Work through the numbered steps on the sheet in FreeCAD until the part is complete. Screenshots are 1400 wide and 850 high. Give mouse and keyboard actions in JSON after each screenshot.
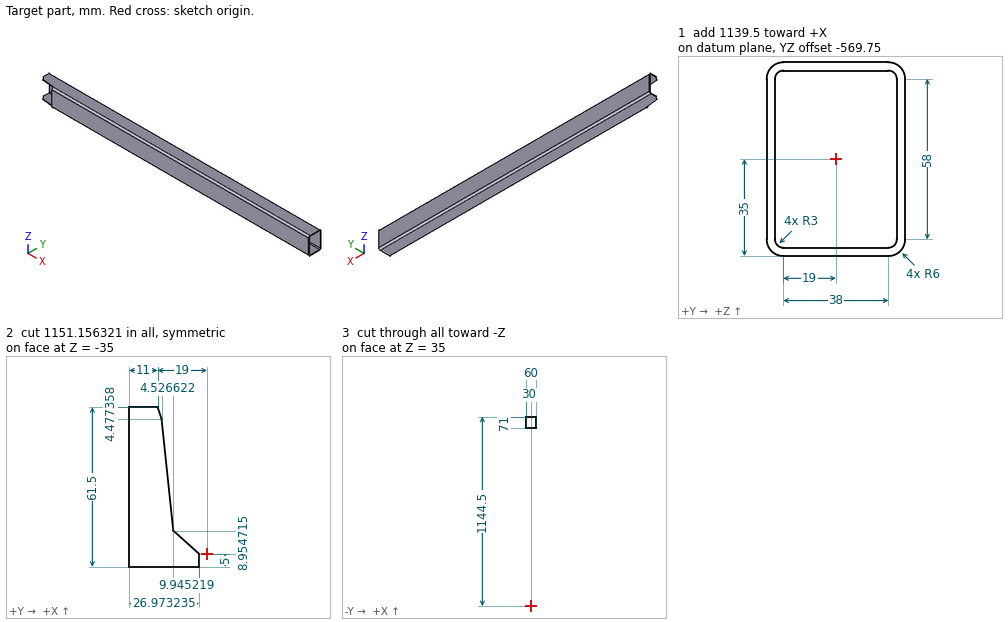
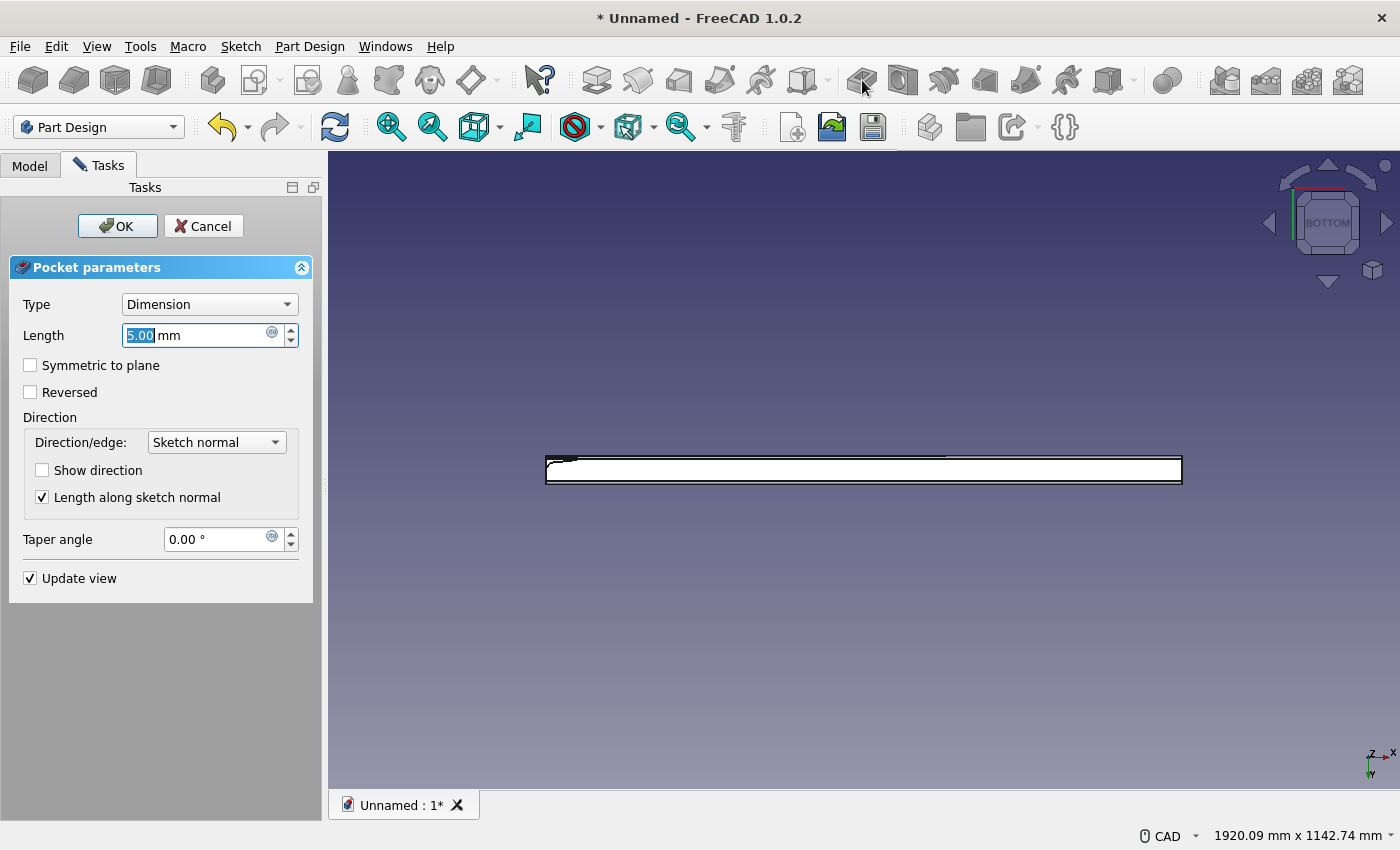
{"action": "type", "text": "1151.156321"}
{"action": "key", "text": "Tab"}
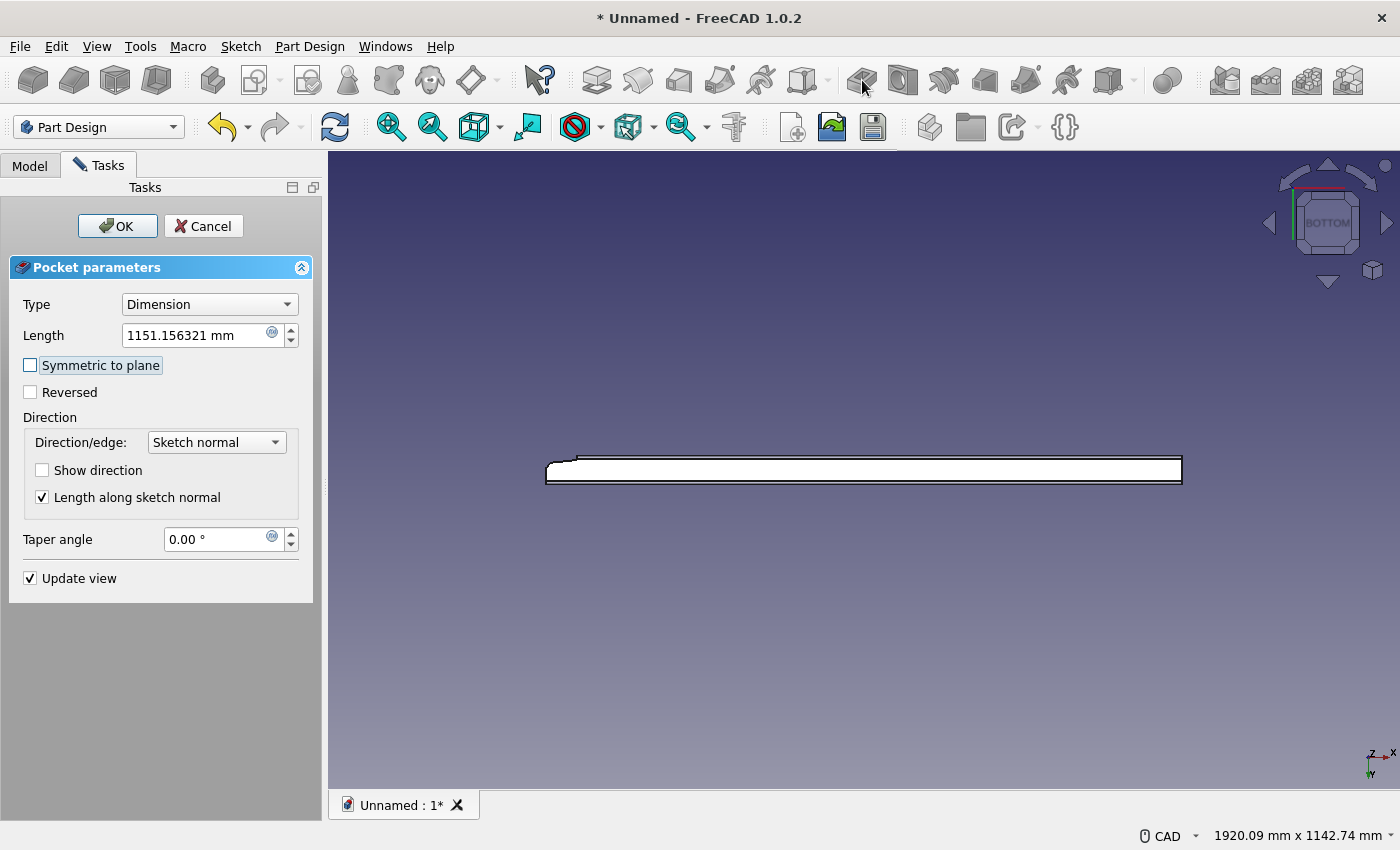
{"action": "left_click", "coordinate": [31, 365]}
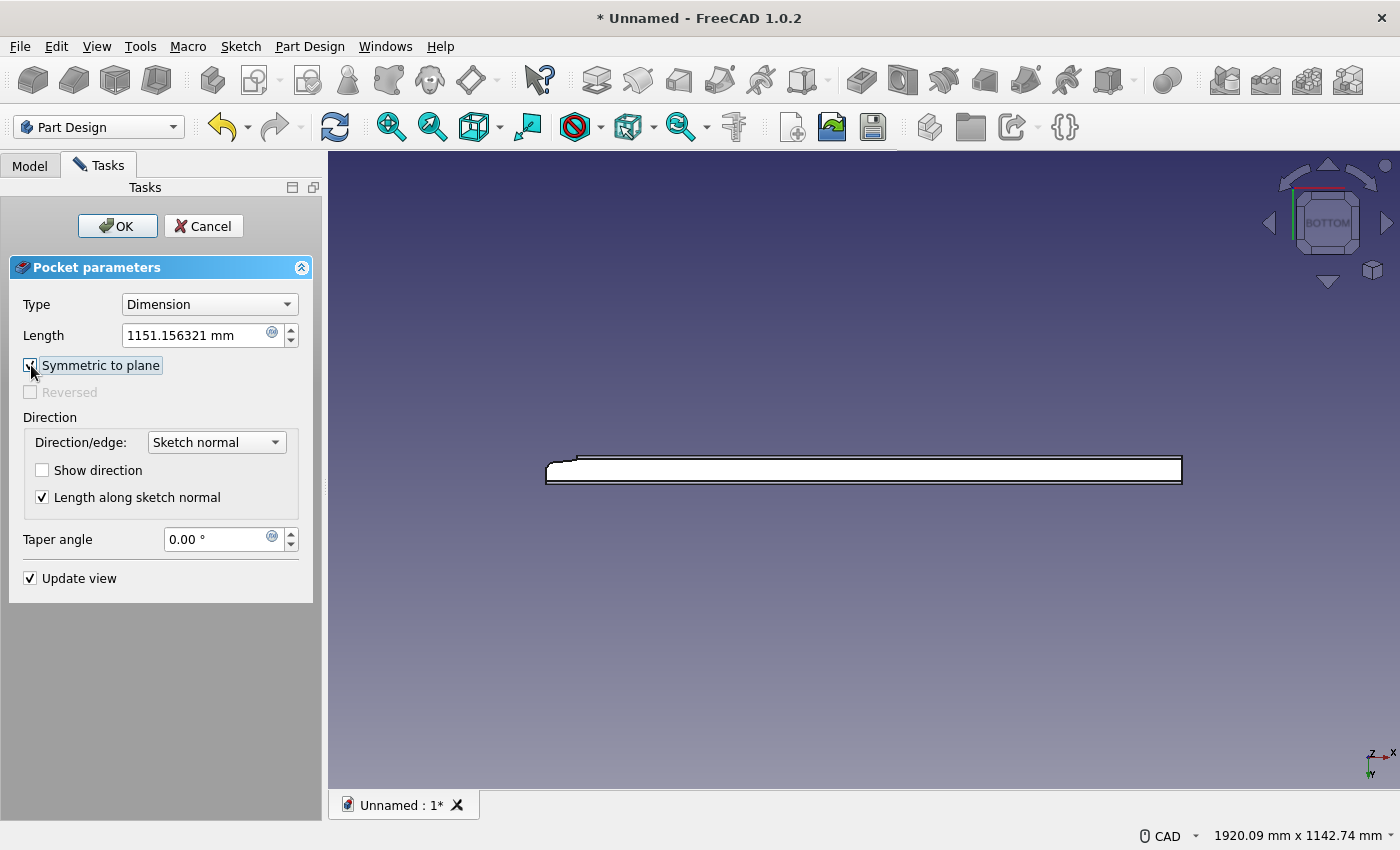
{"action": "left_click", "coordinate": [118, 226]}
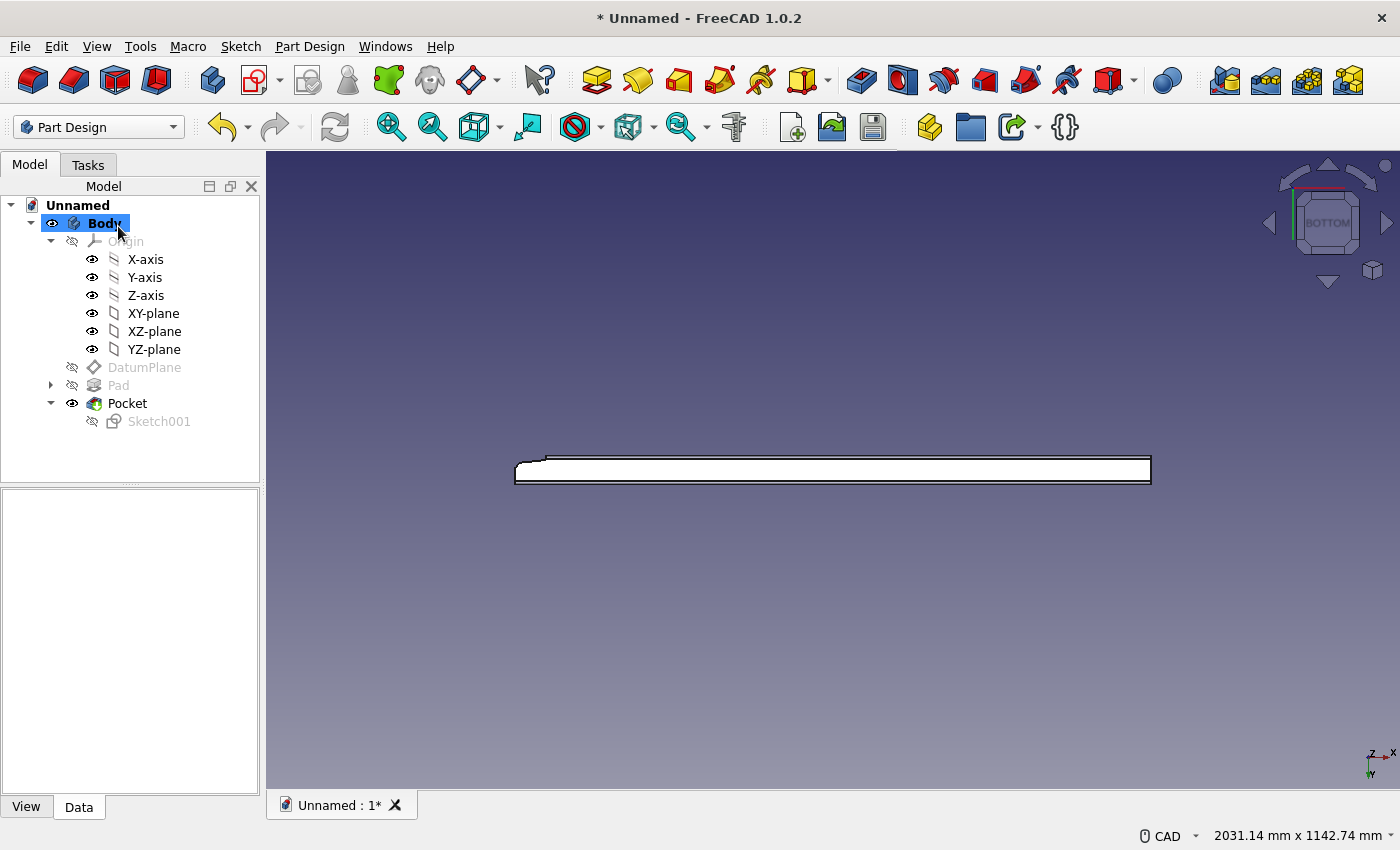
{"action": "key", "text": "0"}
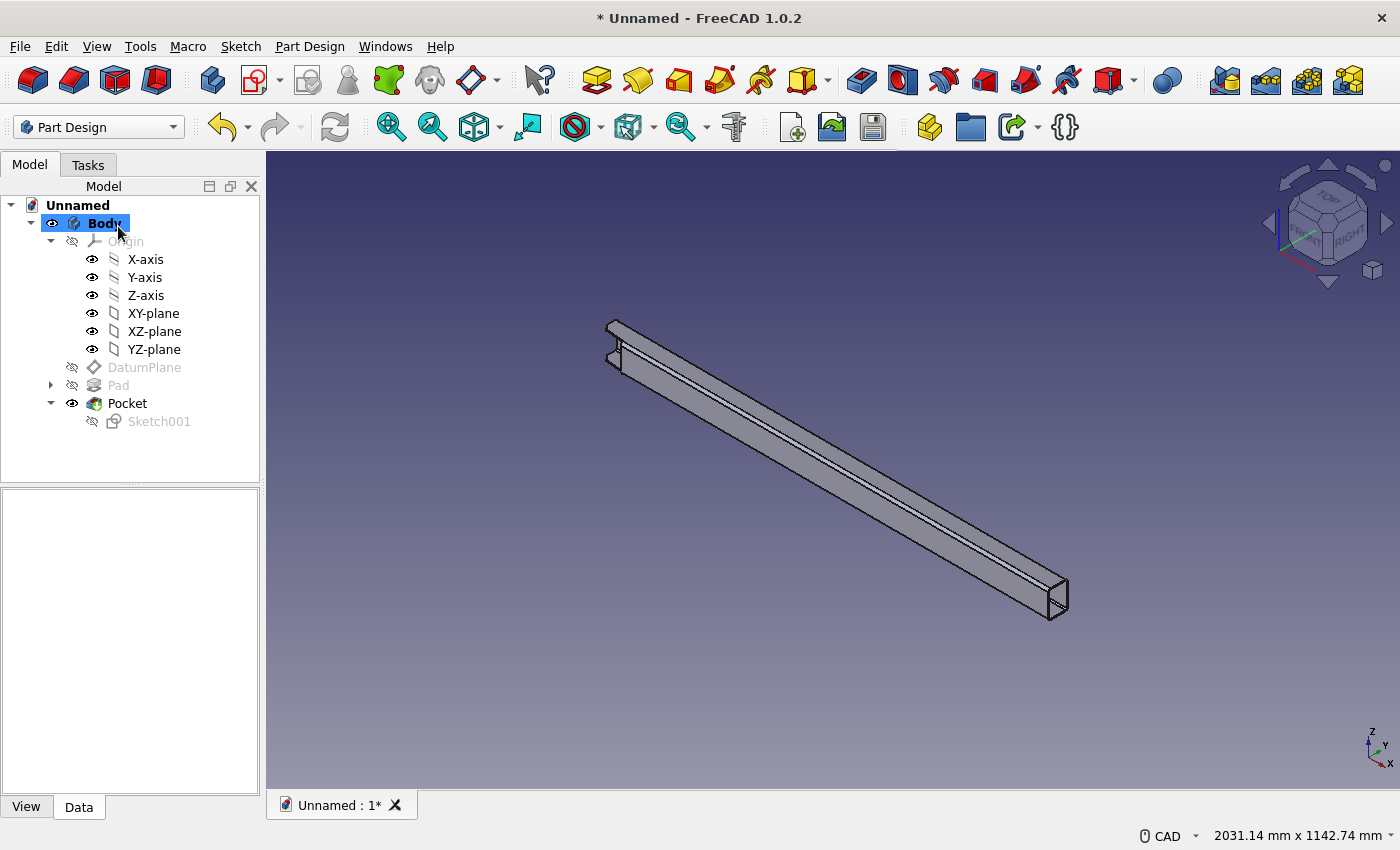
{"action": "left_click", "coordinate": [1028, 563]}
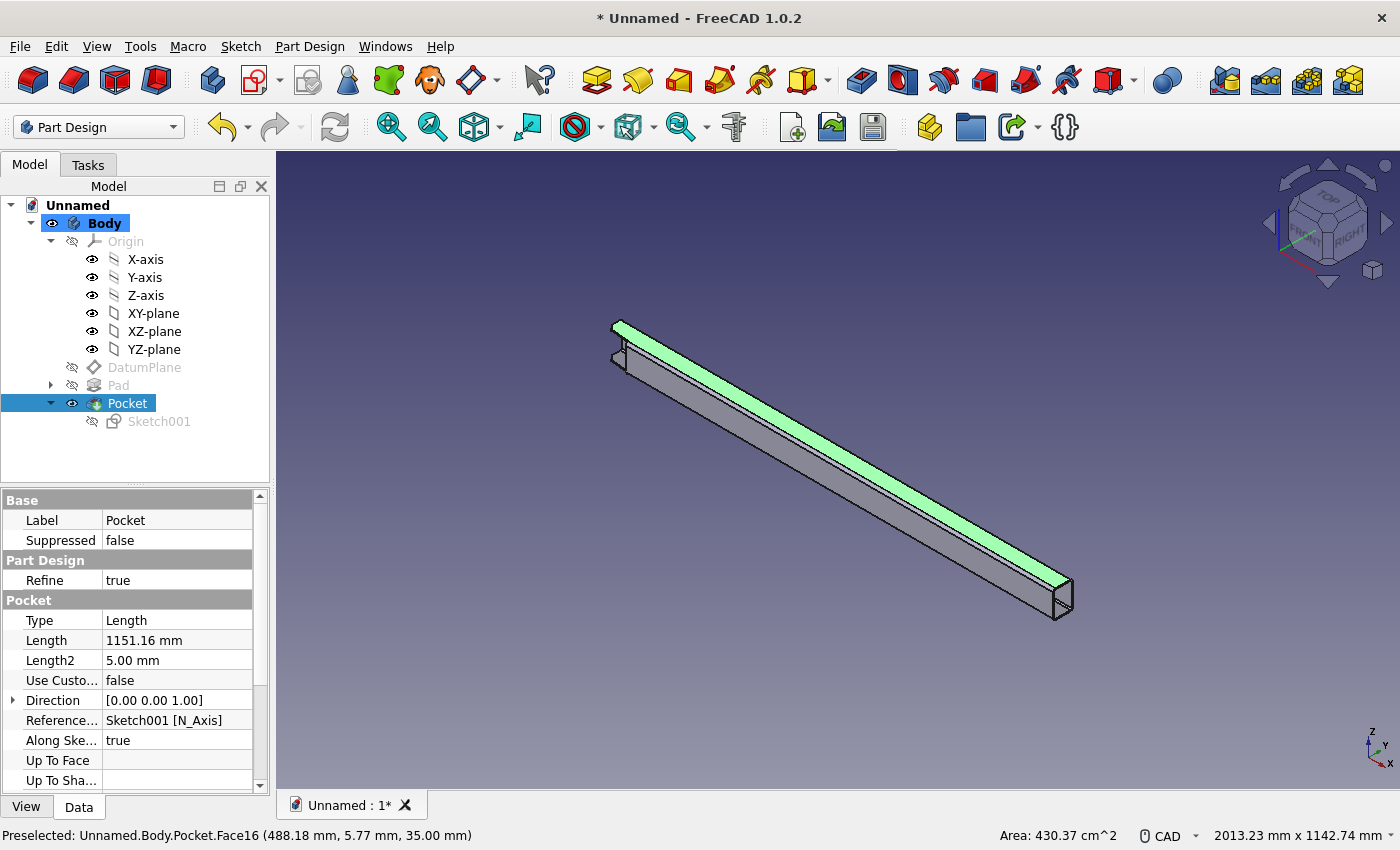
{"action": "left_click", "coordinate": [254, 80]}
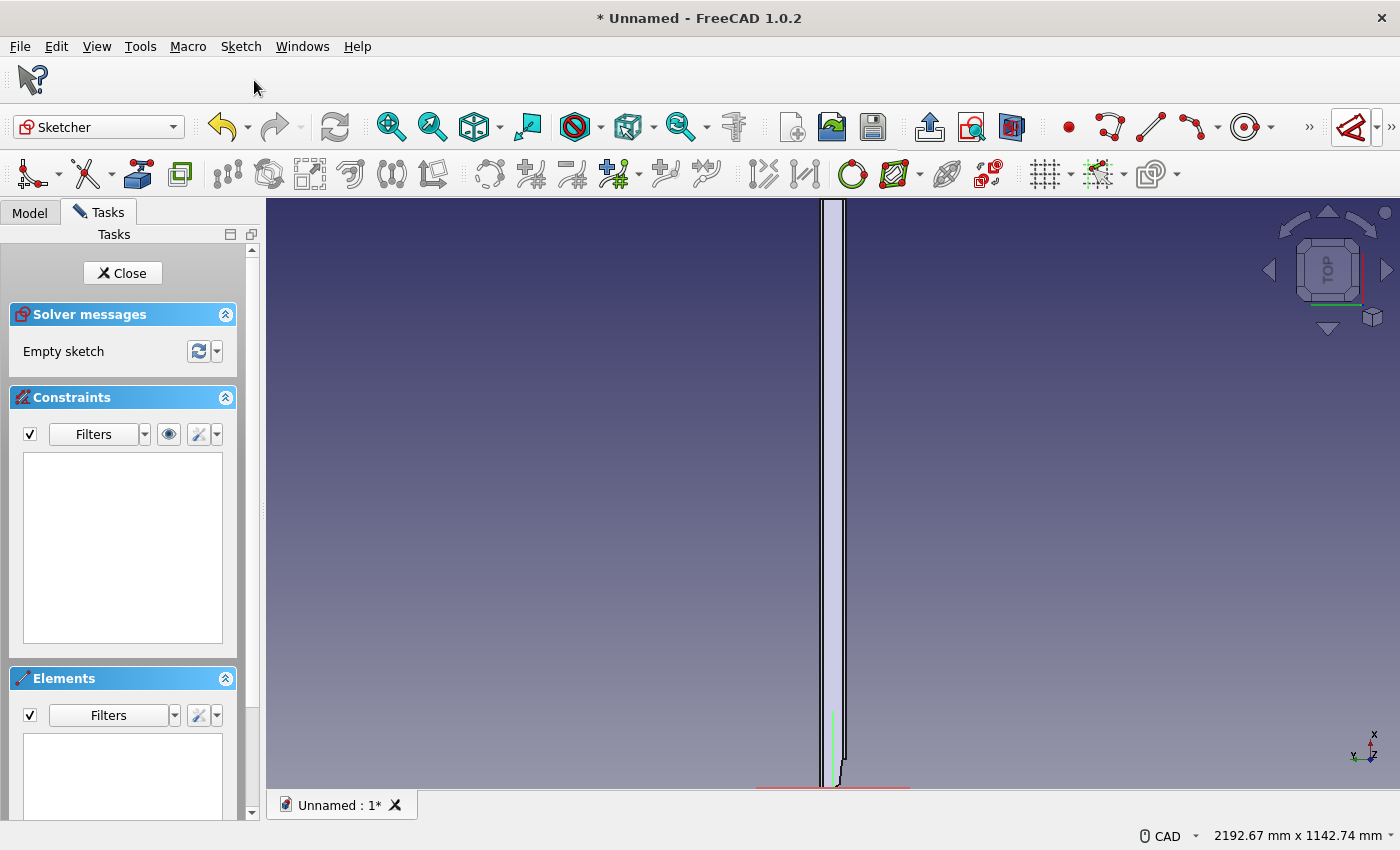
{"action": "scroll", "coordinate": [764, 494], "scroll_direction": "down", "scroll_amount": 5}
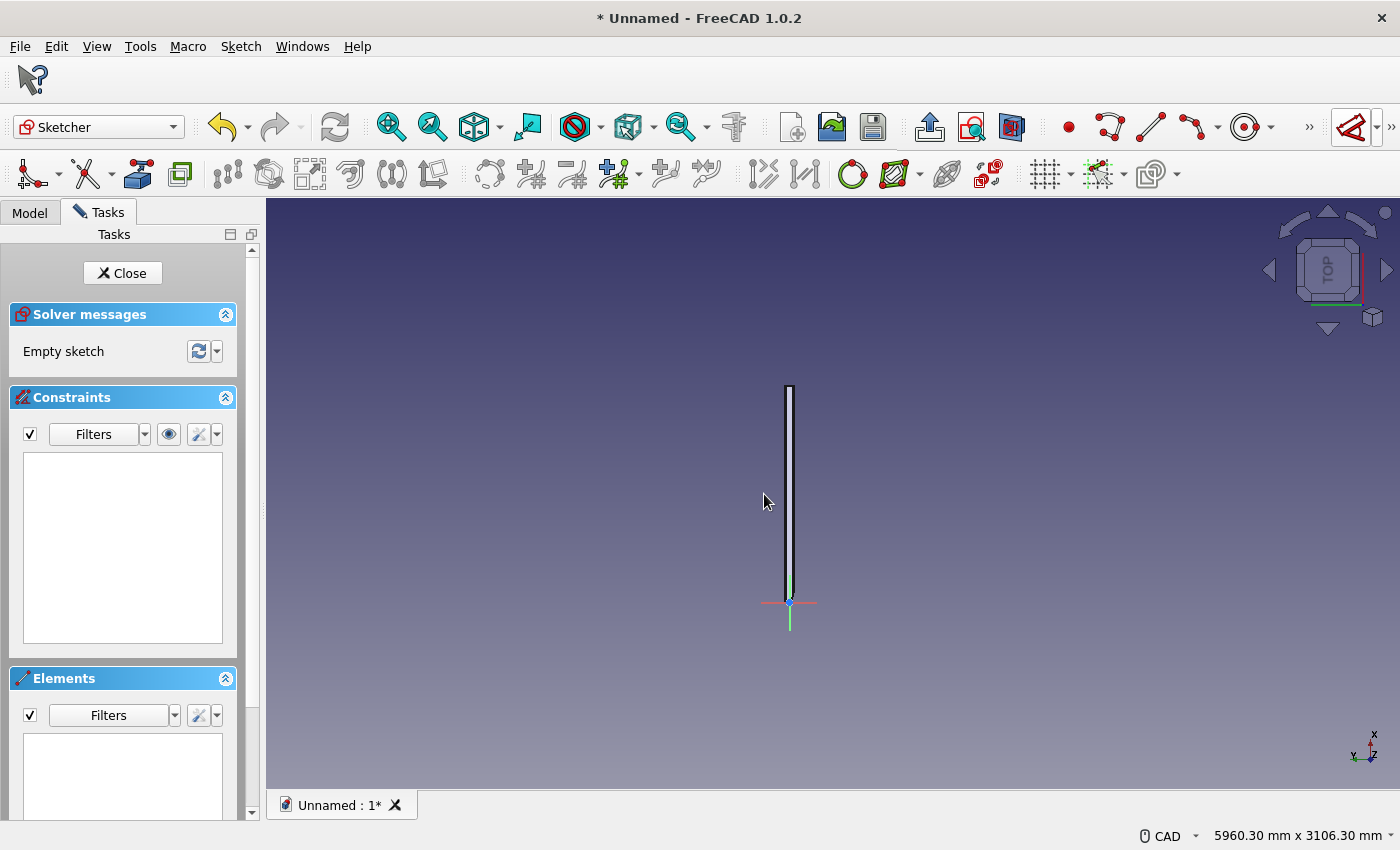
{"action": "scroll", "coordinate": [791, 386], "scroll_direction": "up", "scroll_amount": 15}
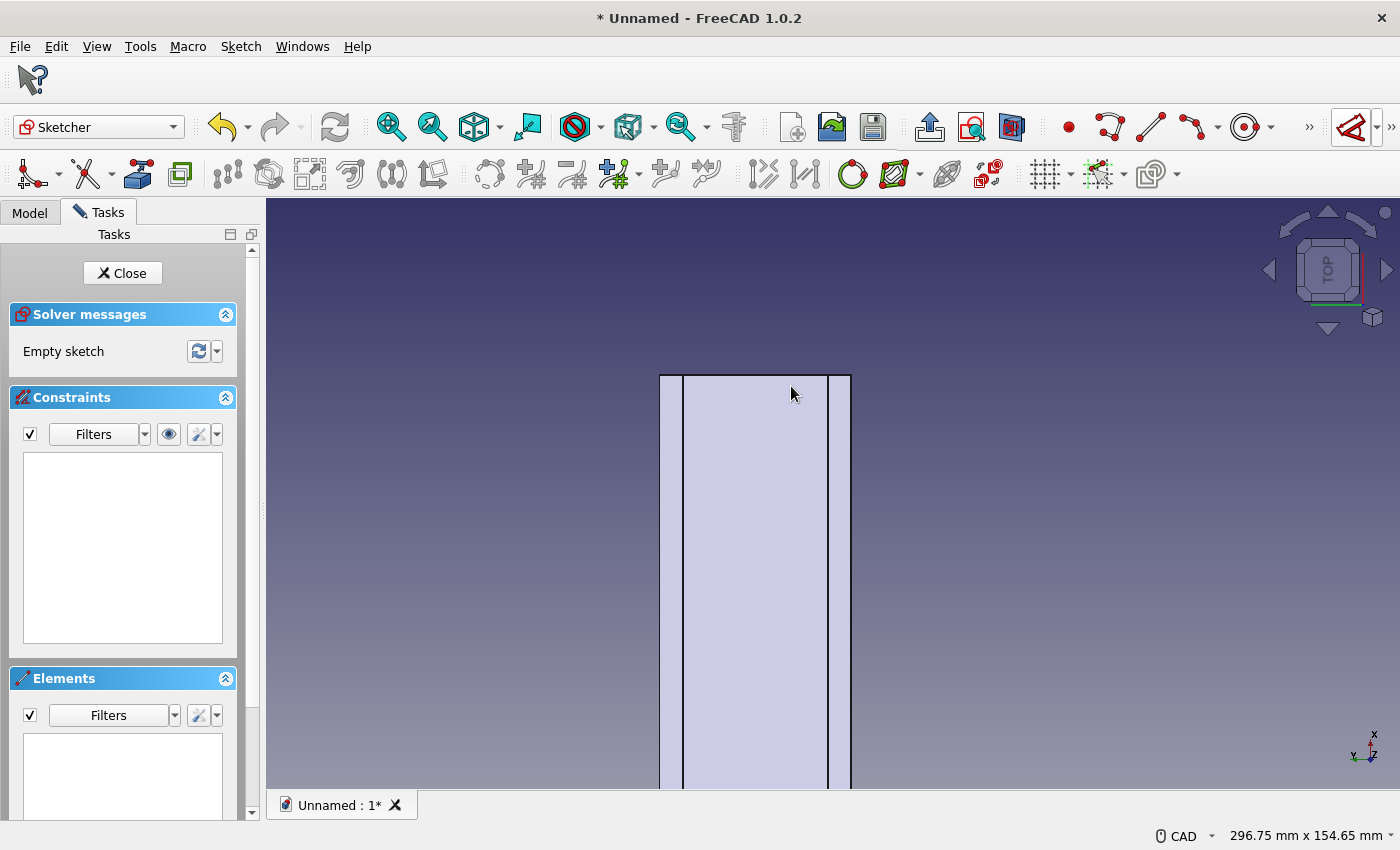
{"action": "scroll", "coordinate": [737, 486], "scroll_direction": "up", "scroll_amount": 2}